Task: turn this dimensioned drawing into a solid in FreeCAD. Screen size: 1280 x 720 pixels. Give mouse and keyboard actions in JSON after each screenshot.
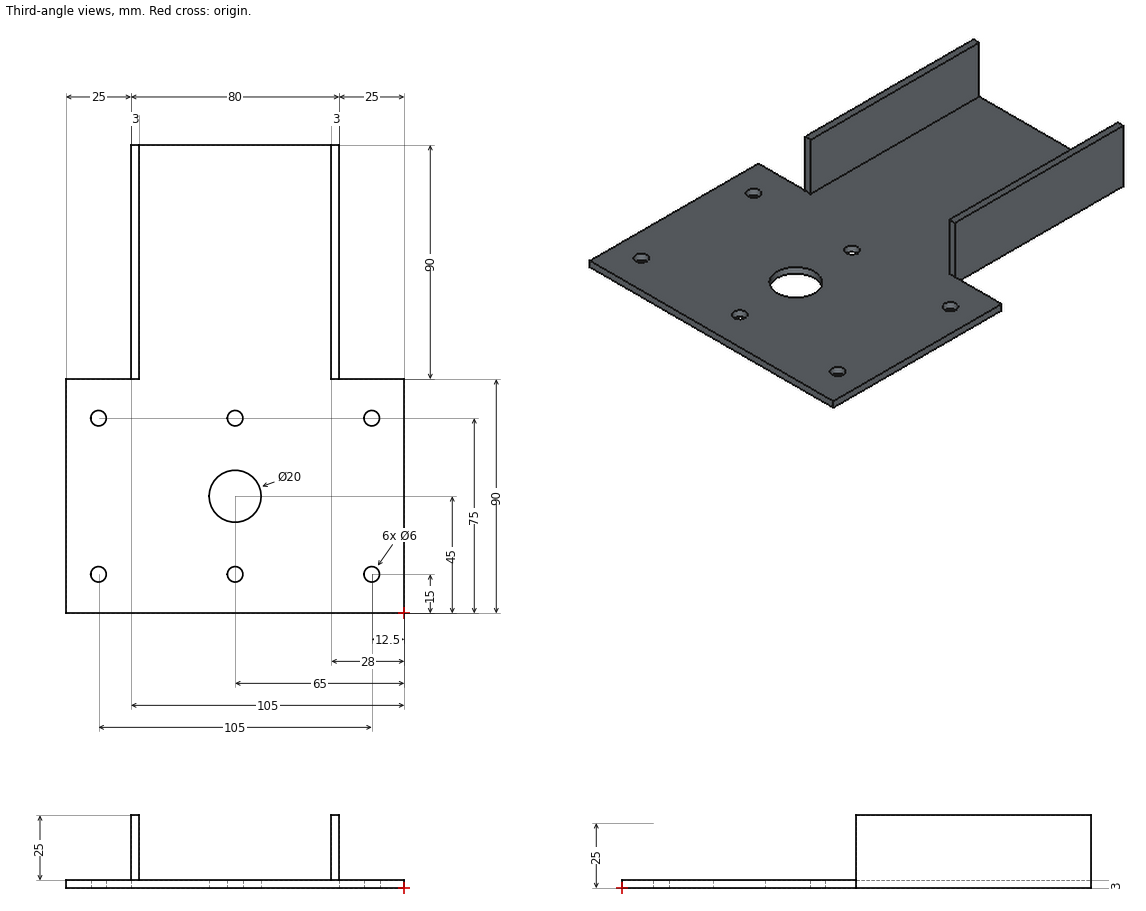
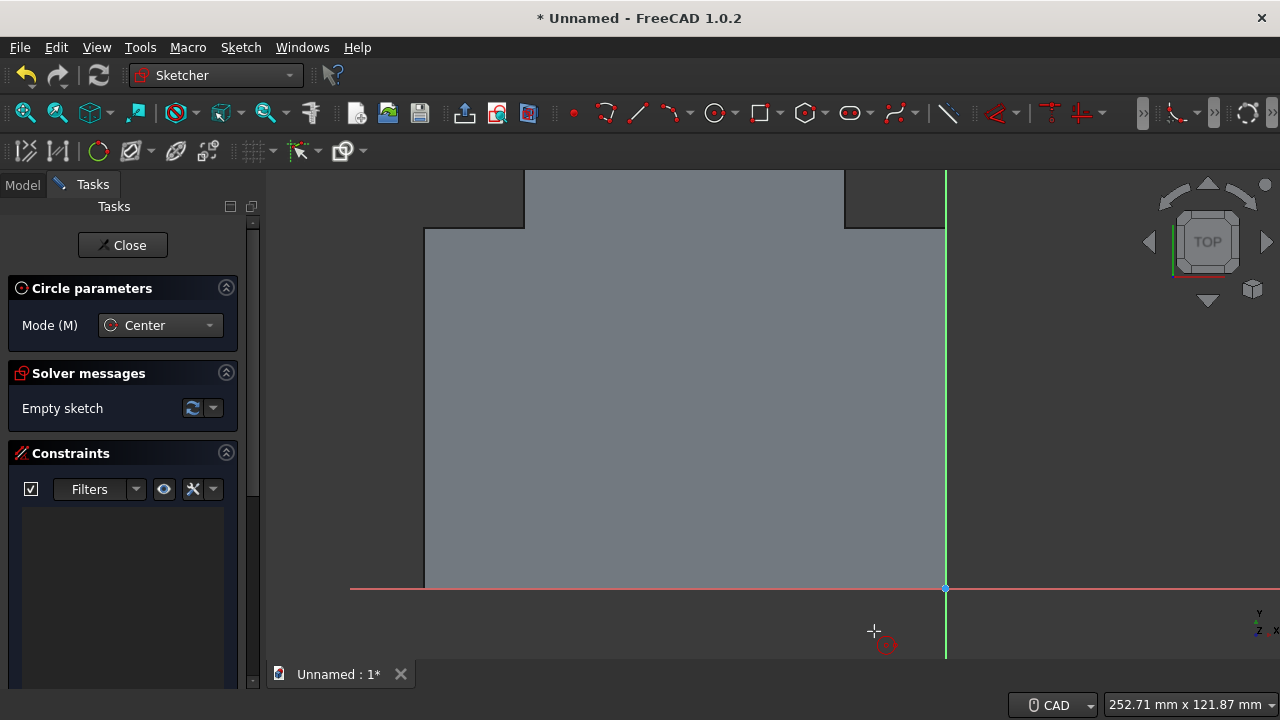
{"action": "left_click", "coordinate": [685, 408]}
{"action": "left_click", "coordinate": [713, 380]}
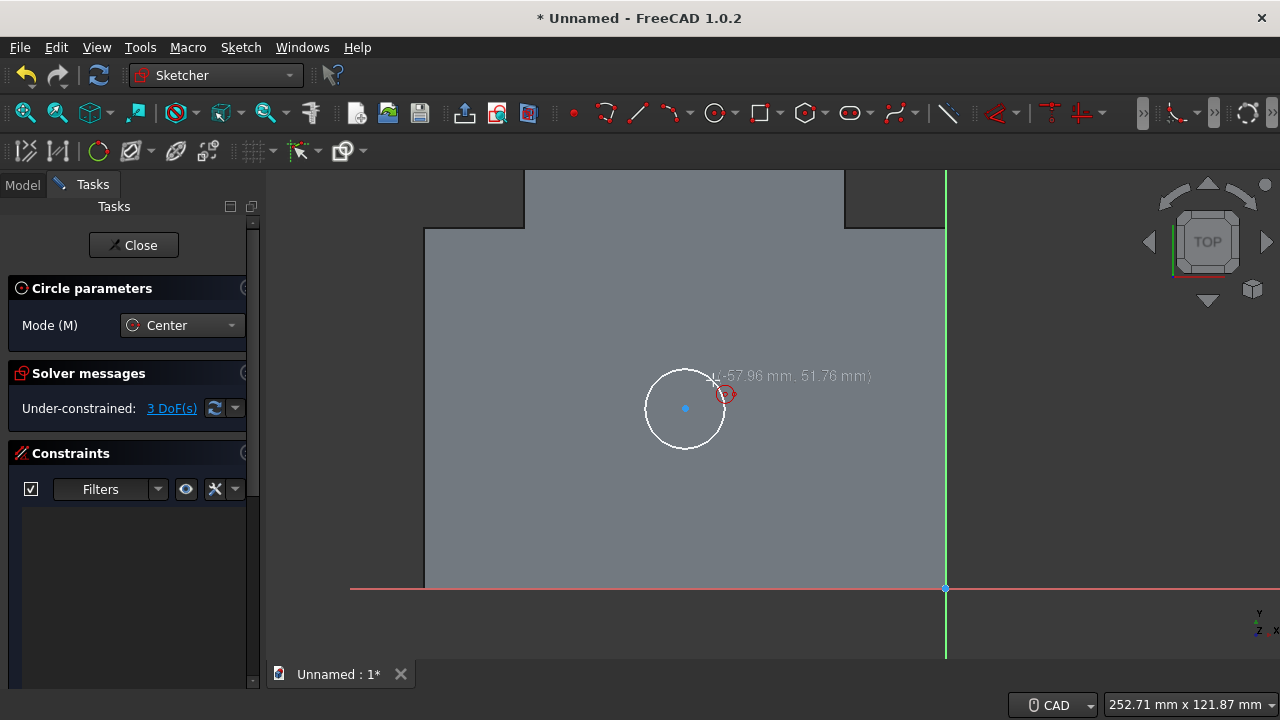
{"action": "scroll", "coordinate": [895, 529], "scroll_direction": "up", "scroll_amount": 4}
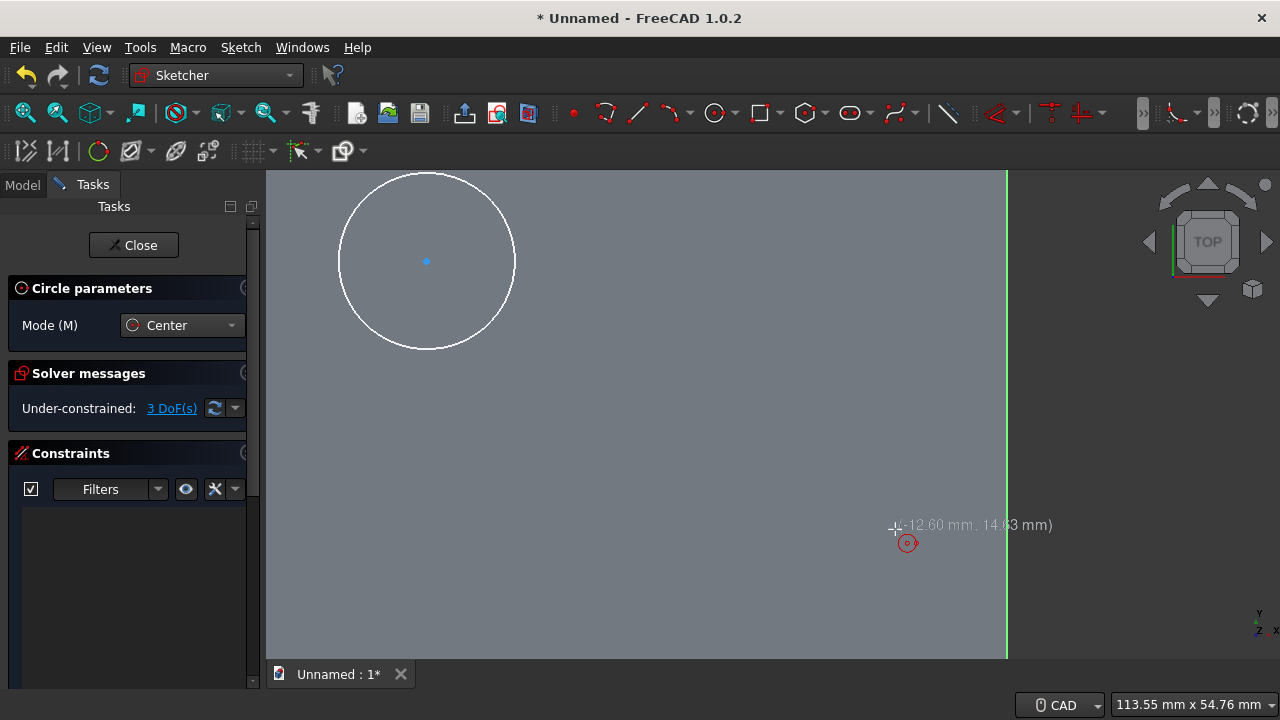
{"action": "left_click", "coordinate": [895, 527]}
{"action": "left_click", "coordinate": [914, 508]}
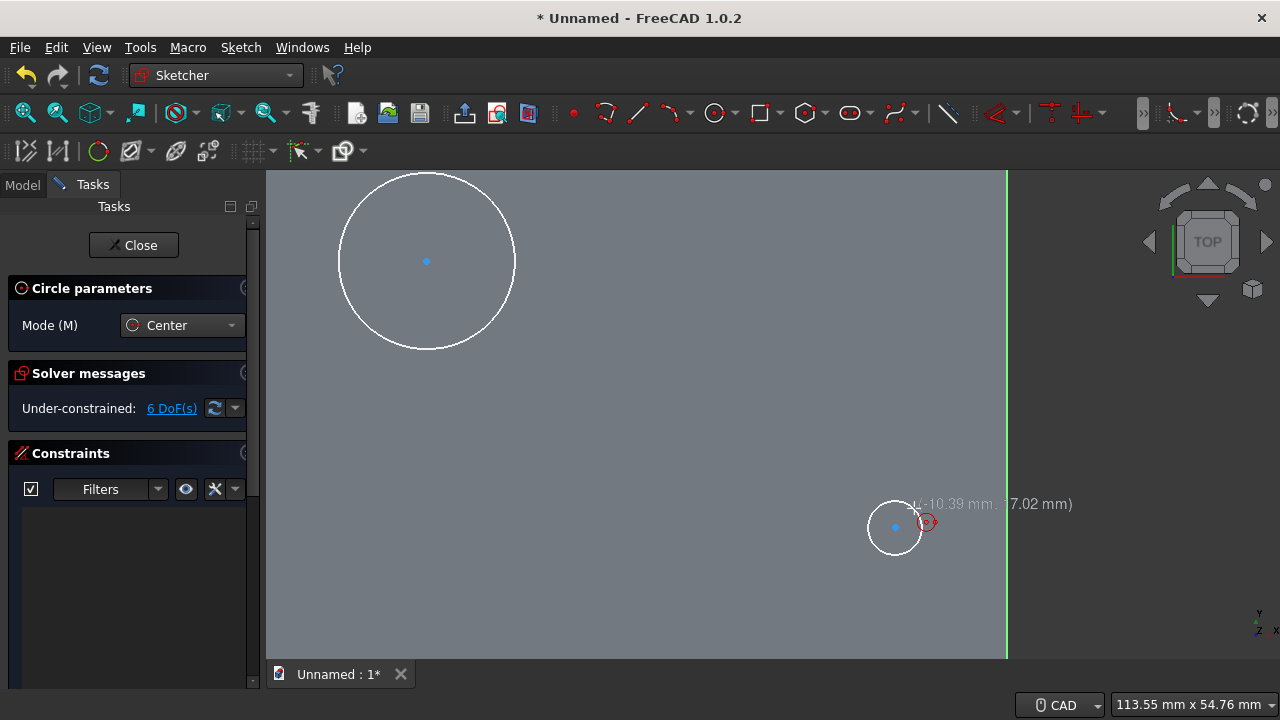
{"action": "left_click", "coordinate": [426, 527]}
{"action": "left_click", "coordinate": [445, 508]}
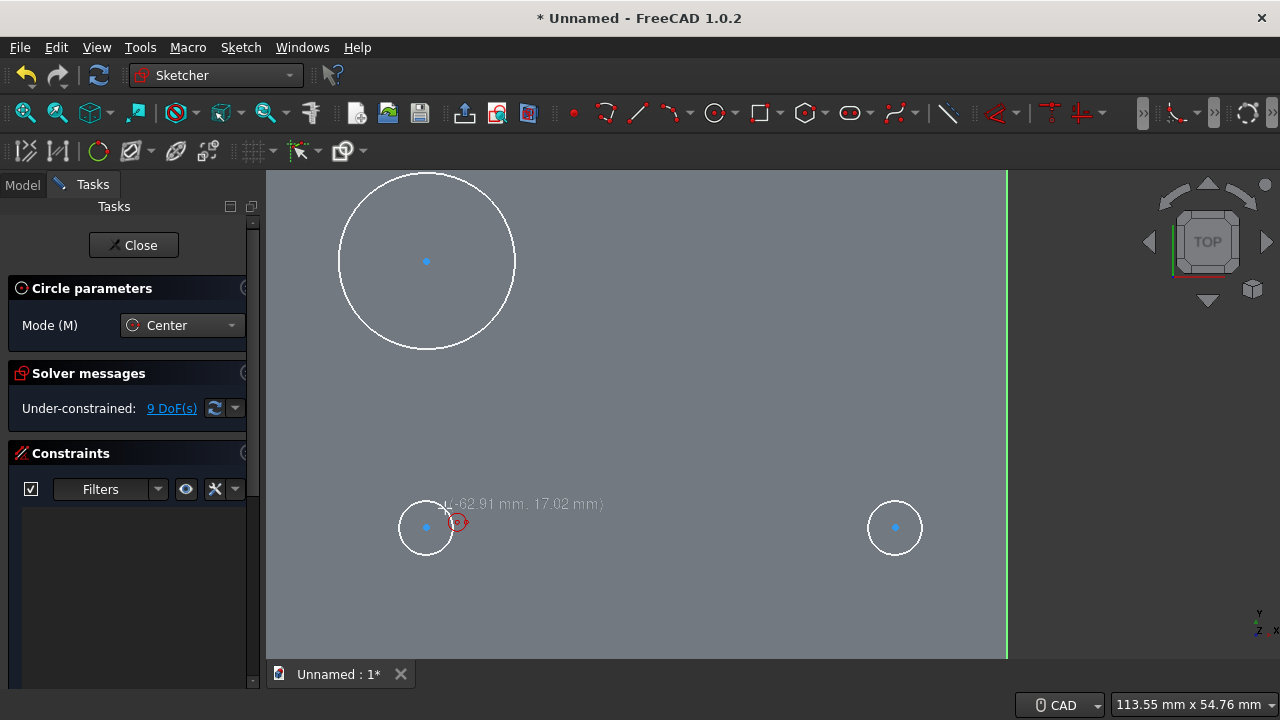
{"action": "scroll", "coordinate": [897, 498], "scroll_direction": "down", "scroll_amount": 4}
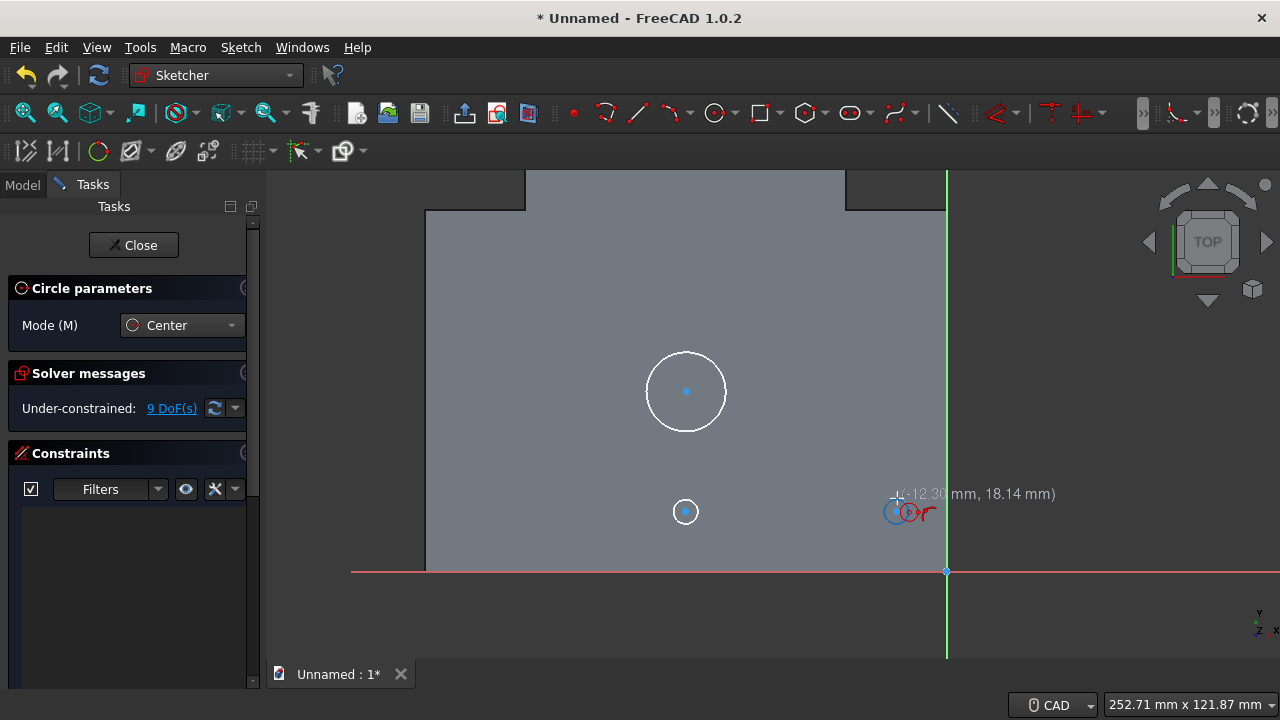
{"action": "scroll", "coordinate": [475, 511], "scroll_direction": "up", "scroll_amount": 4}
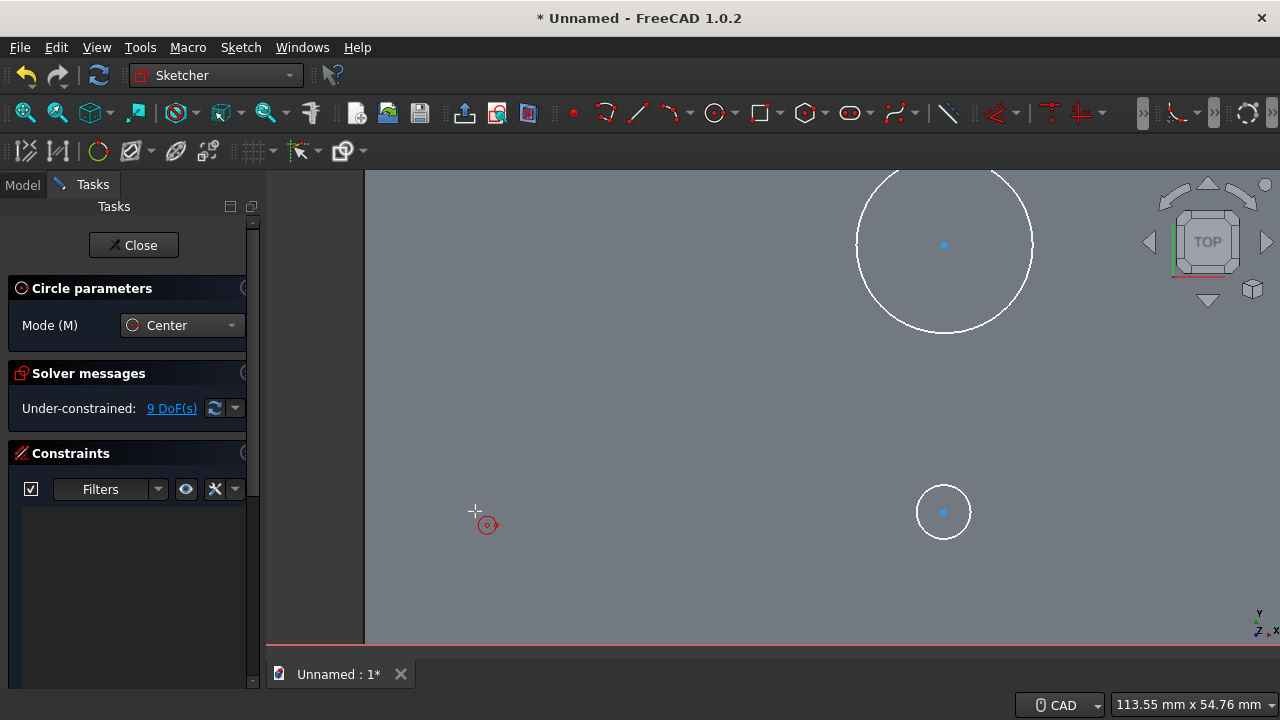
{"action": "left_click", "coordinate": [475, 511]}
{"action": "left_click", "coordinate": [494, 492]}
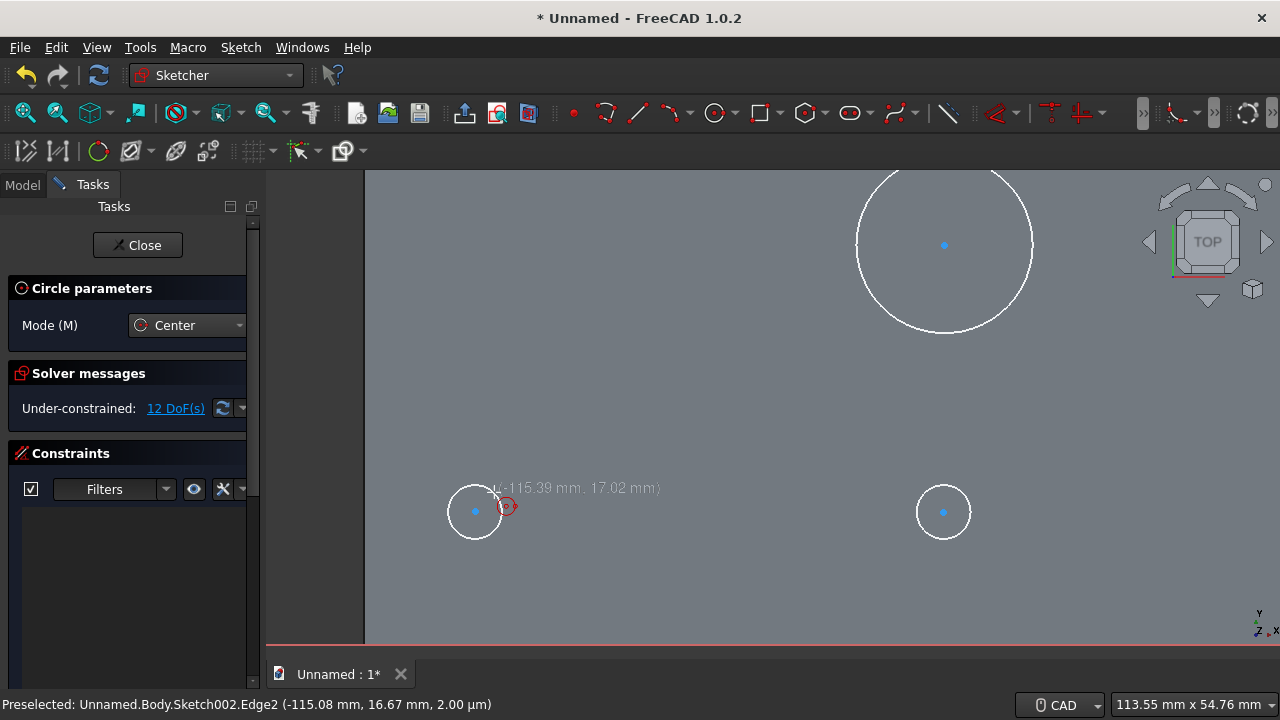
{"action": "scroll", "coordinate": [474, 511], "scroll_direction": "down", "scroll_amount": 4}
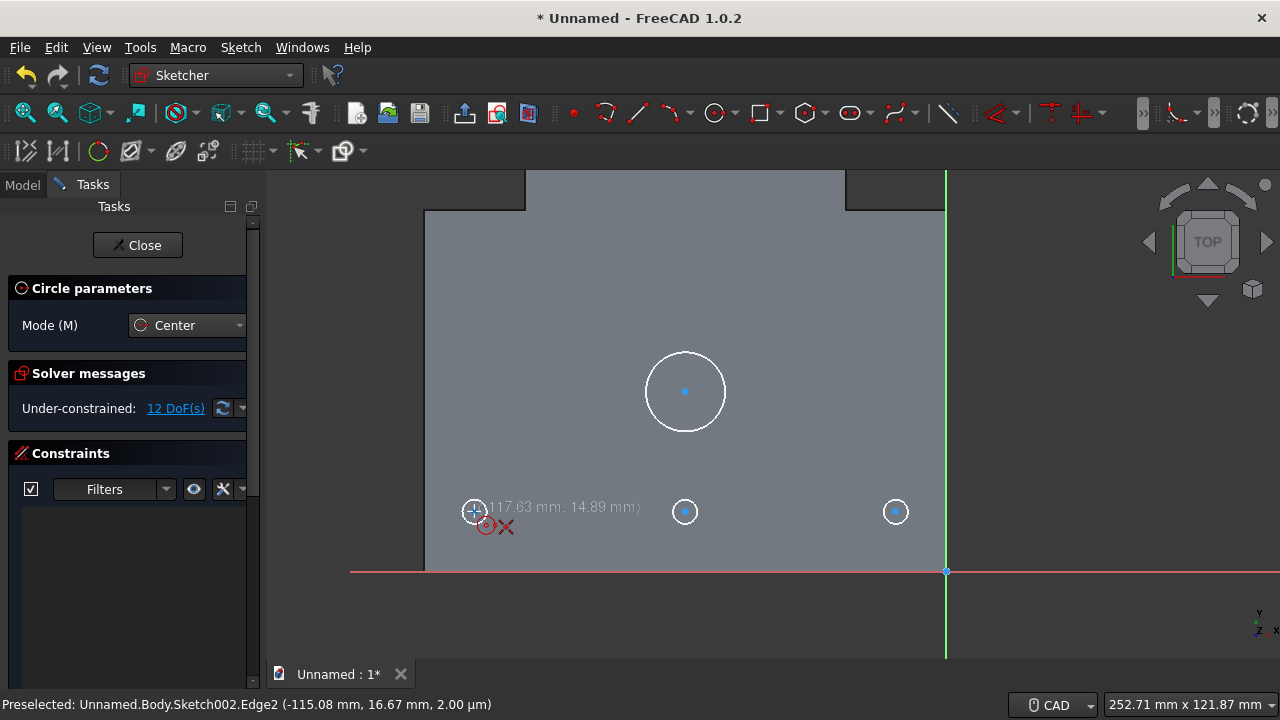
{"action": "scroll", "coordinate": [475, 271], "scroll_direction": "up", "scroll_amount": 4}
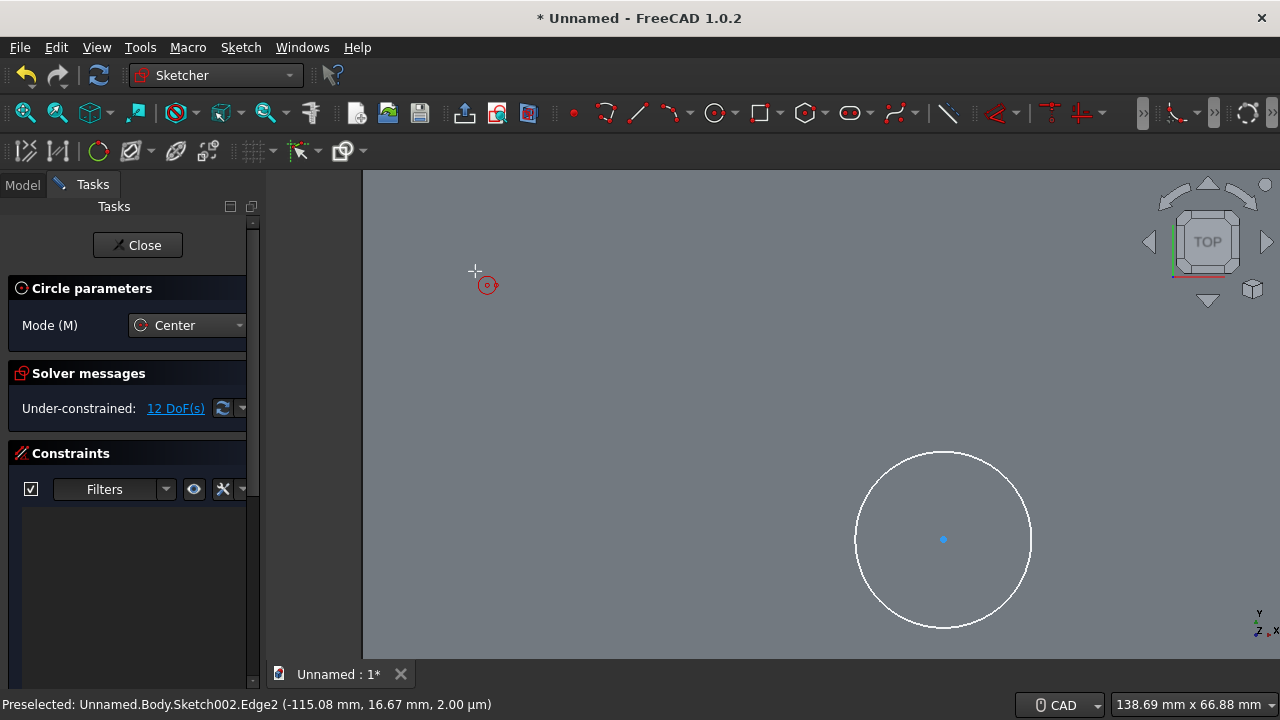
{"action": "left_click", "coordinate": [474, 270]}
{"action": "left_click", "coordinate": [493, 251]}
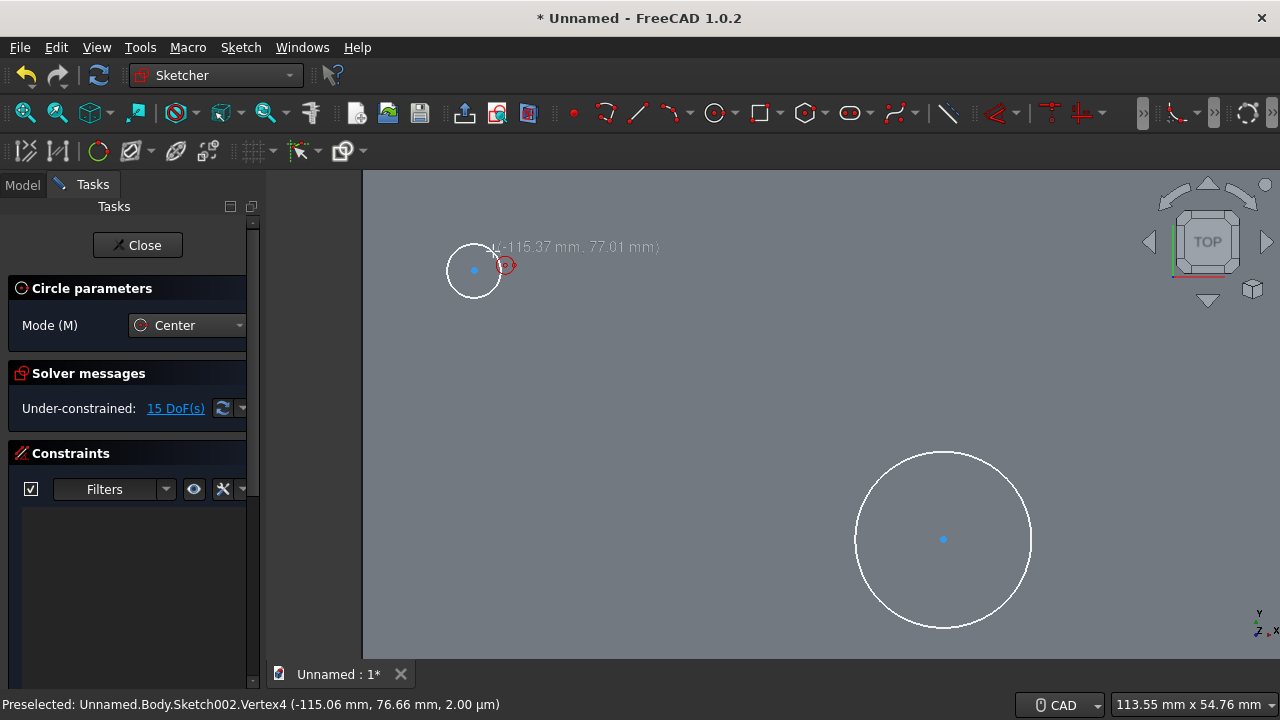
{"action": "left_click", "coordinate": [943, 270]}
{"action": "left_click", "coordinate": [962, 251]}